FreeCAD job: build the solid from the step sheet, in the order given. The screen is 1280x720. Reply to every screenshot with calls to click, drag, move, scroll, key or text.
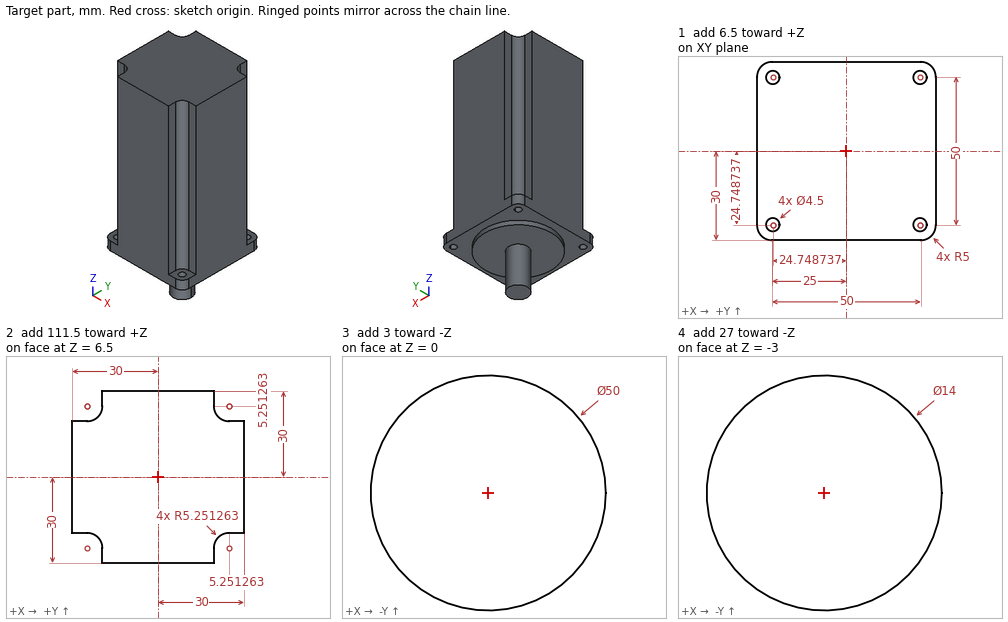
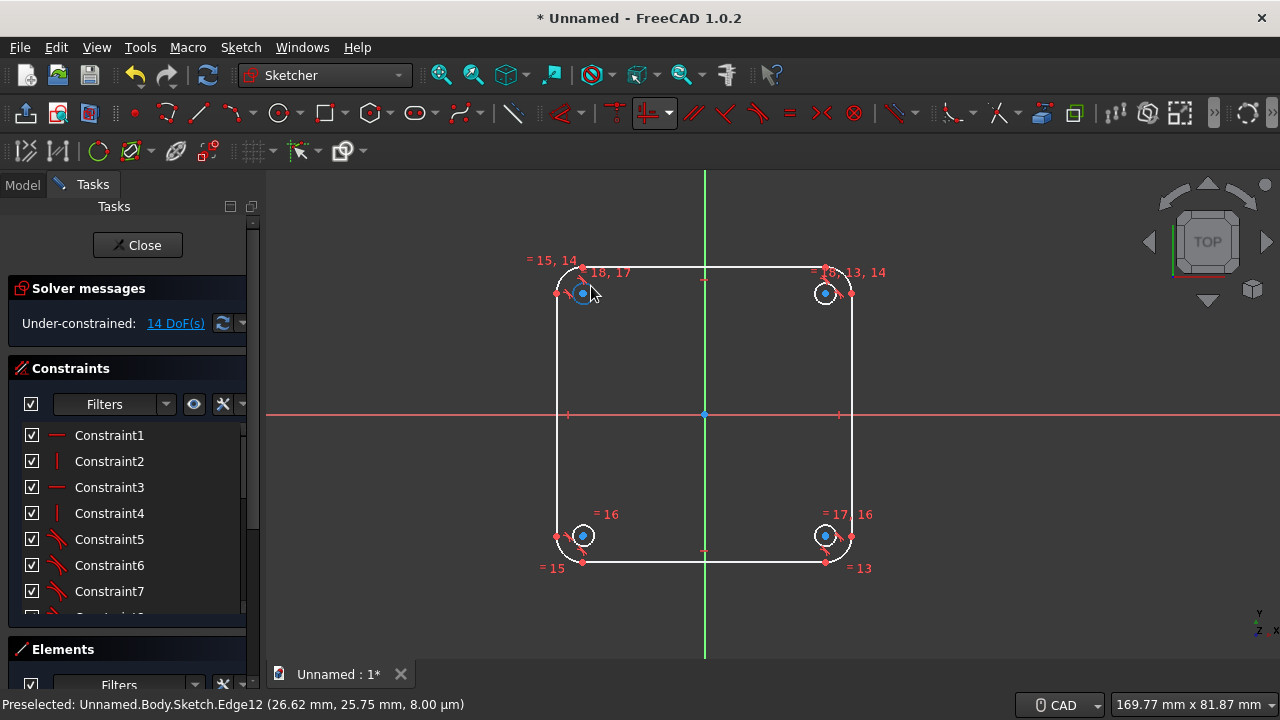
scroll(584, 536, up, 13)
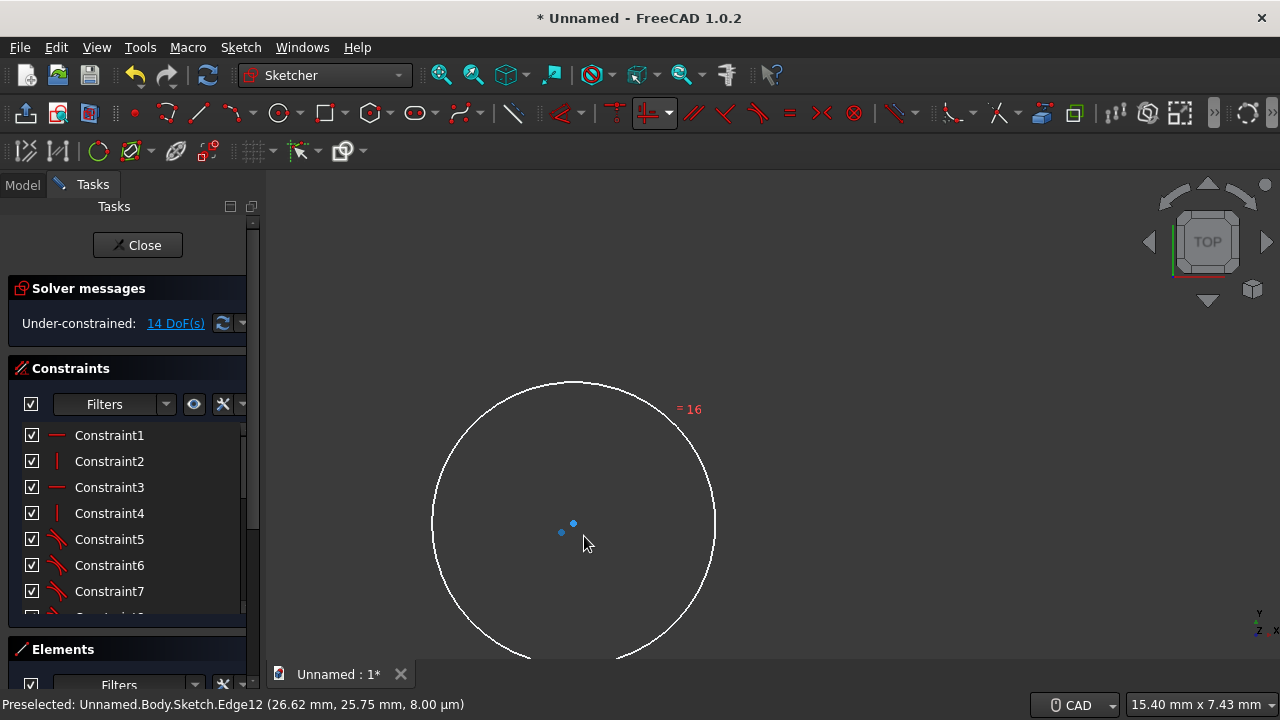
click(574, 524)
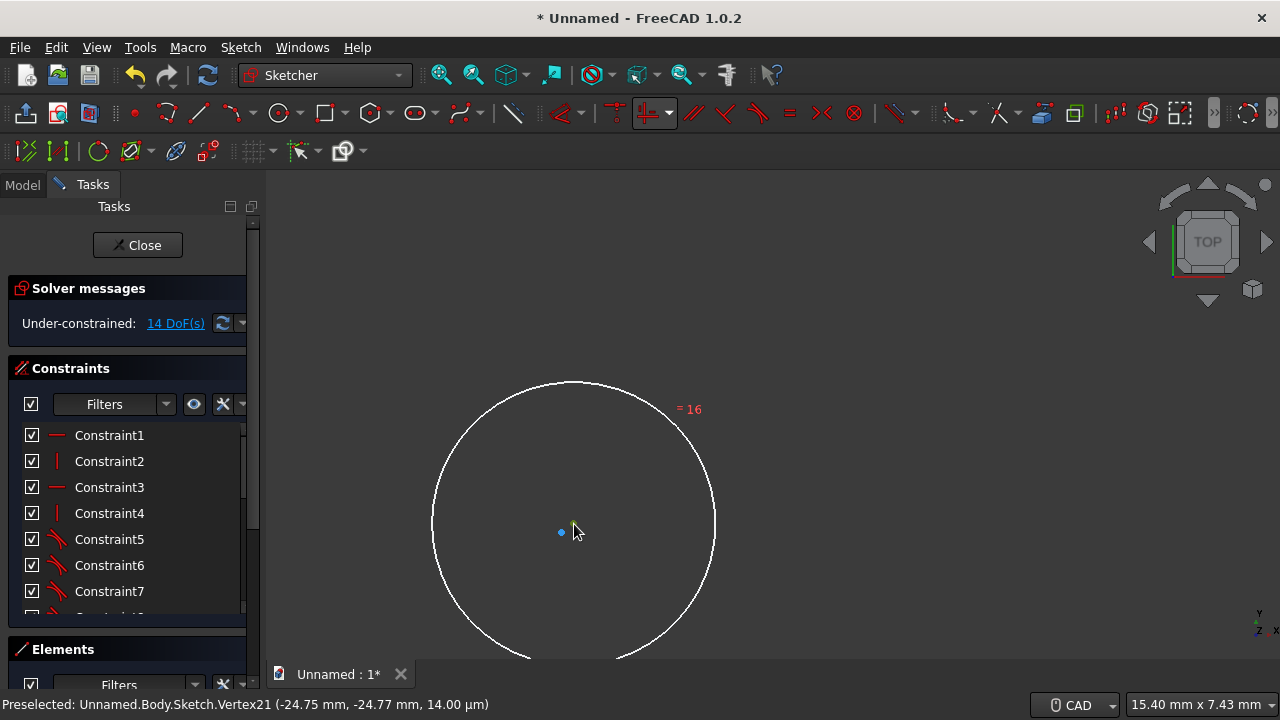
scroll(584, 537, down, 13)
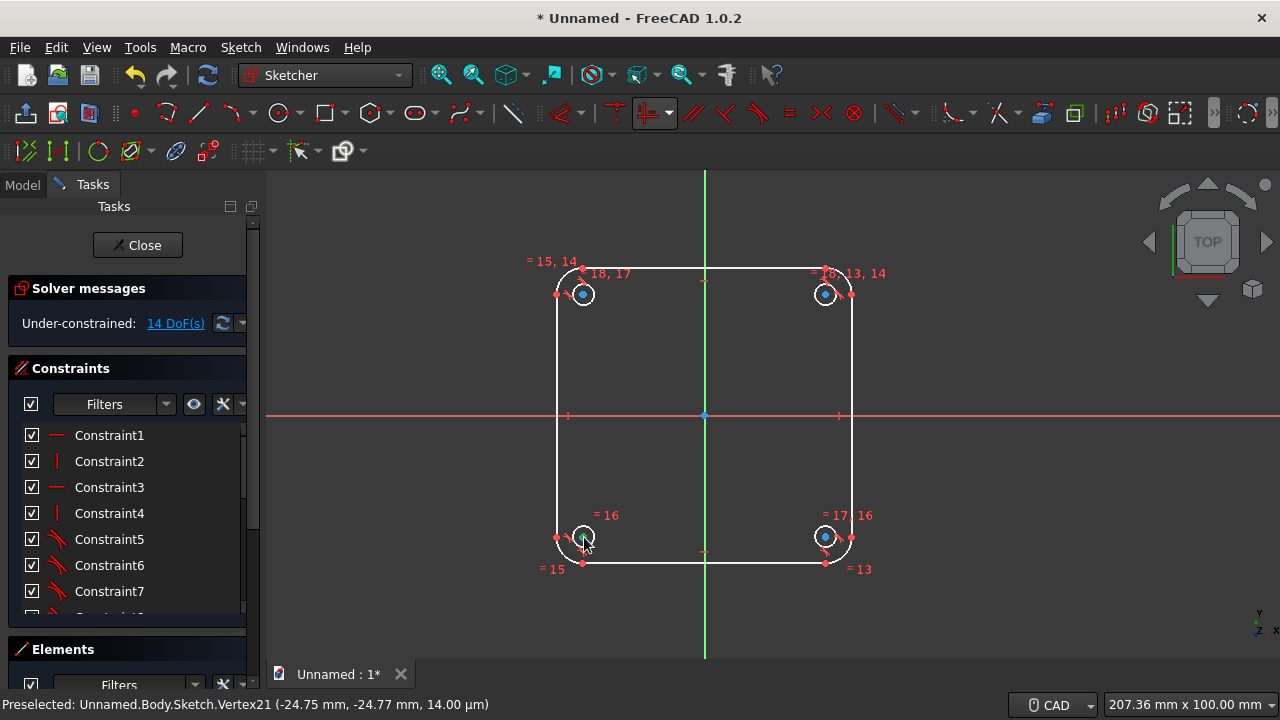
scroll(826, 537, up, 14)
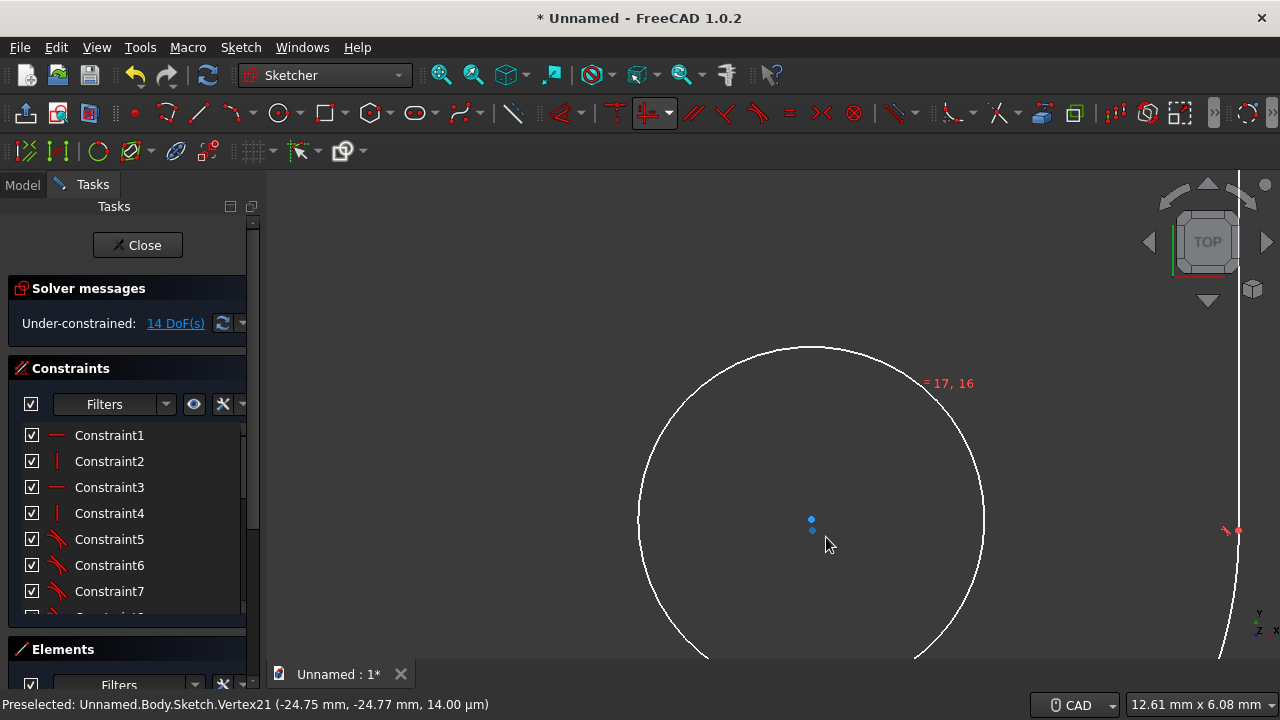
click(811, 520)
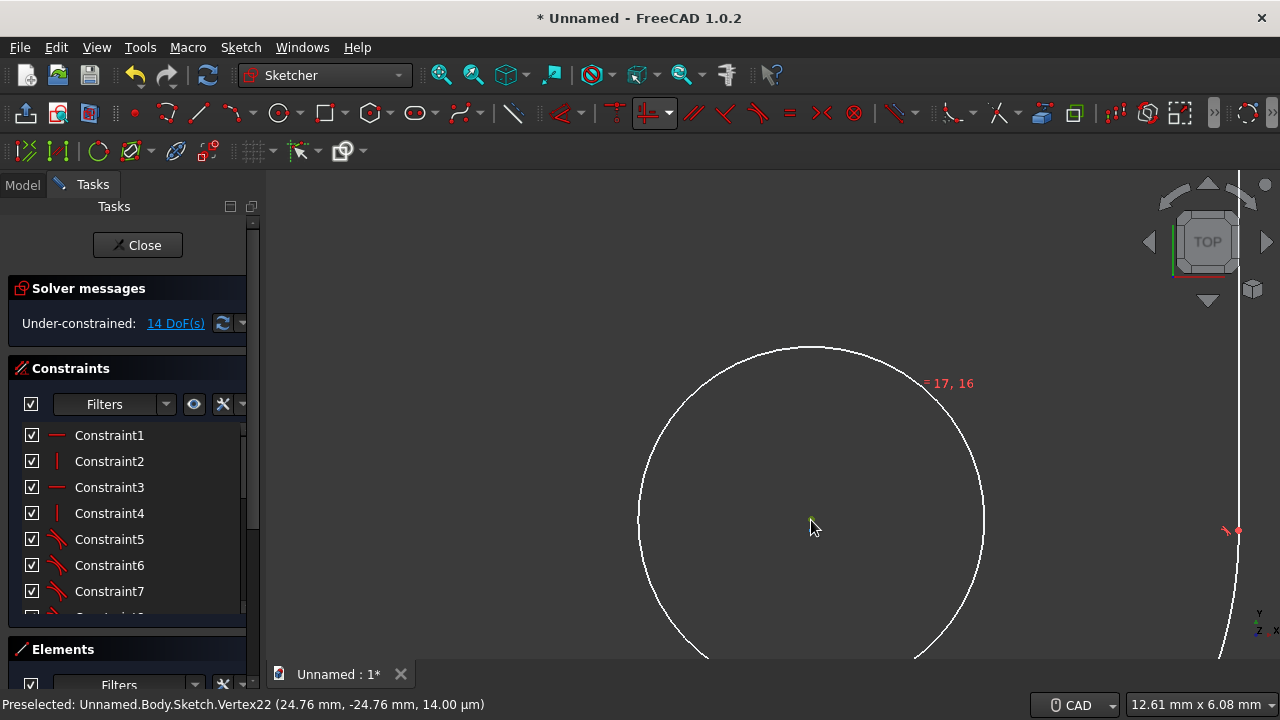
scroll(826, 537, down, 14)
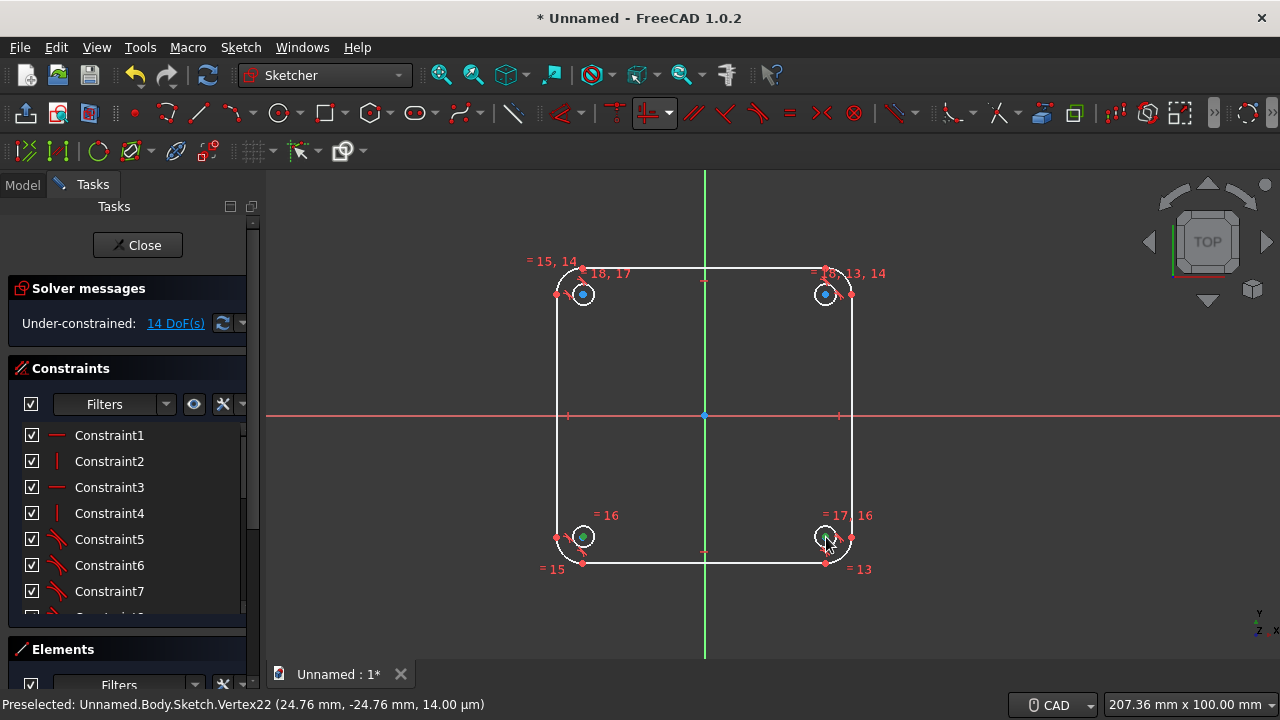
click(705, 600)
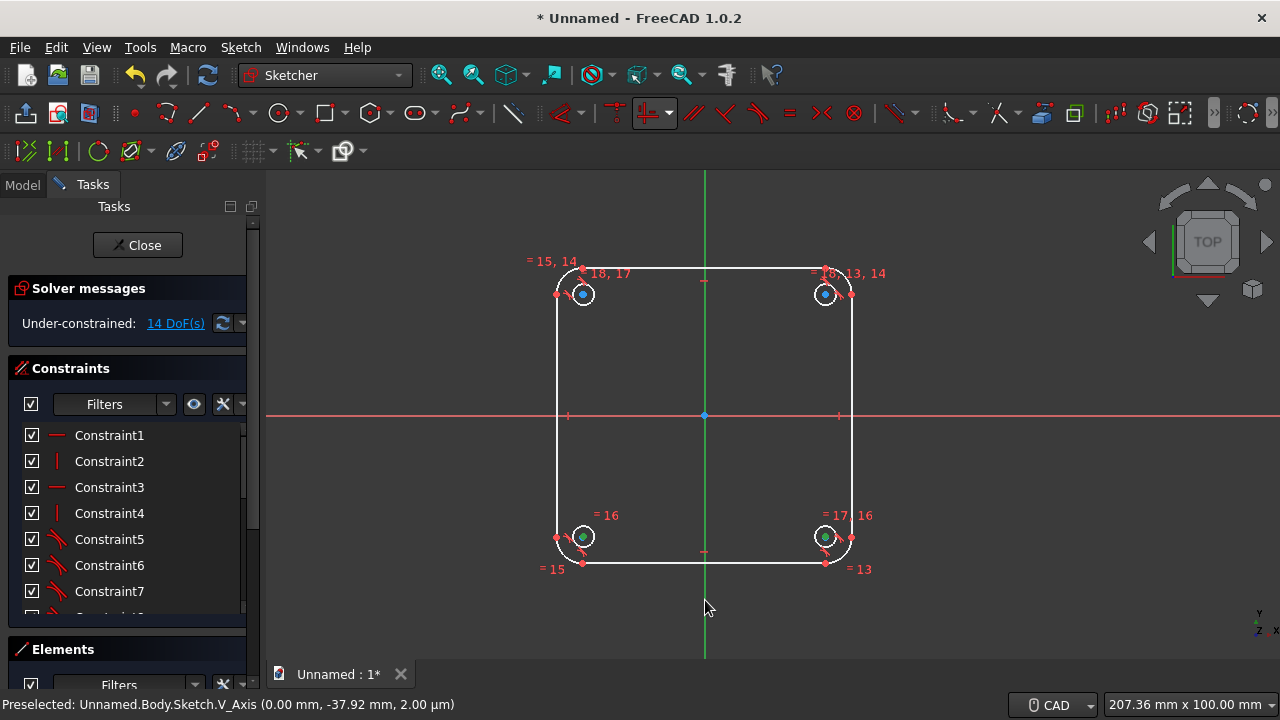
key(s)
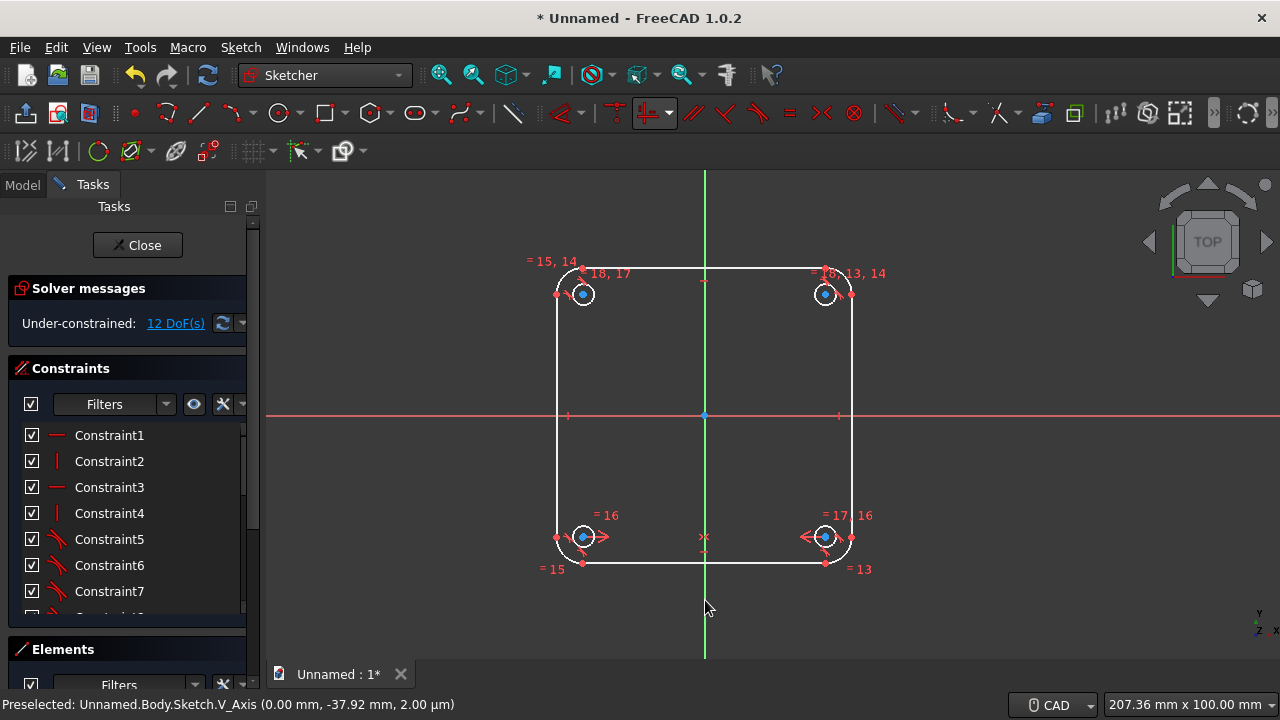
scroll(584, 537, up, 12)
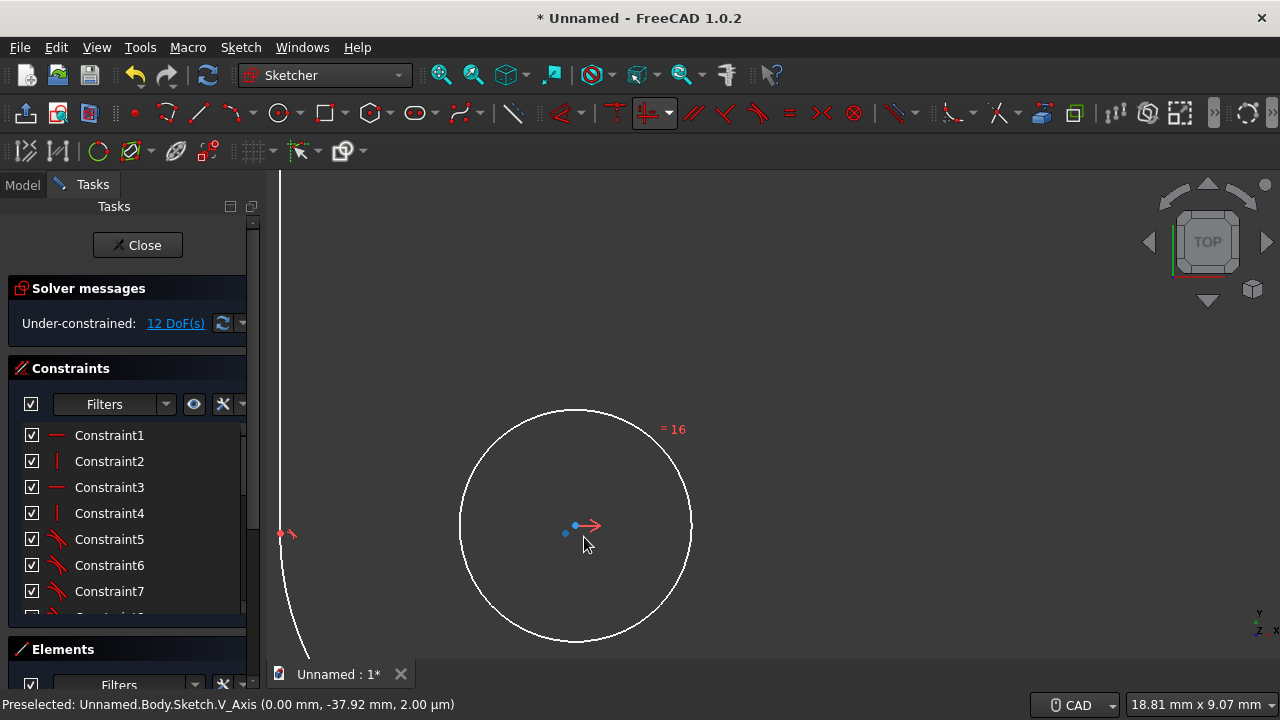
click(576, 526)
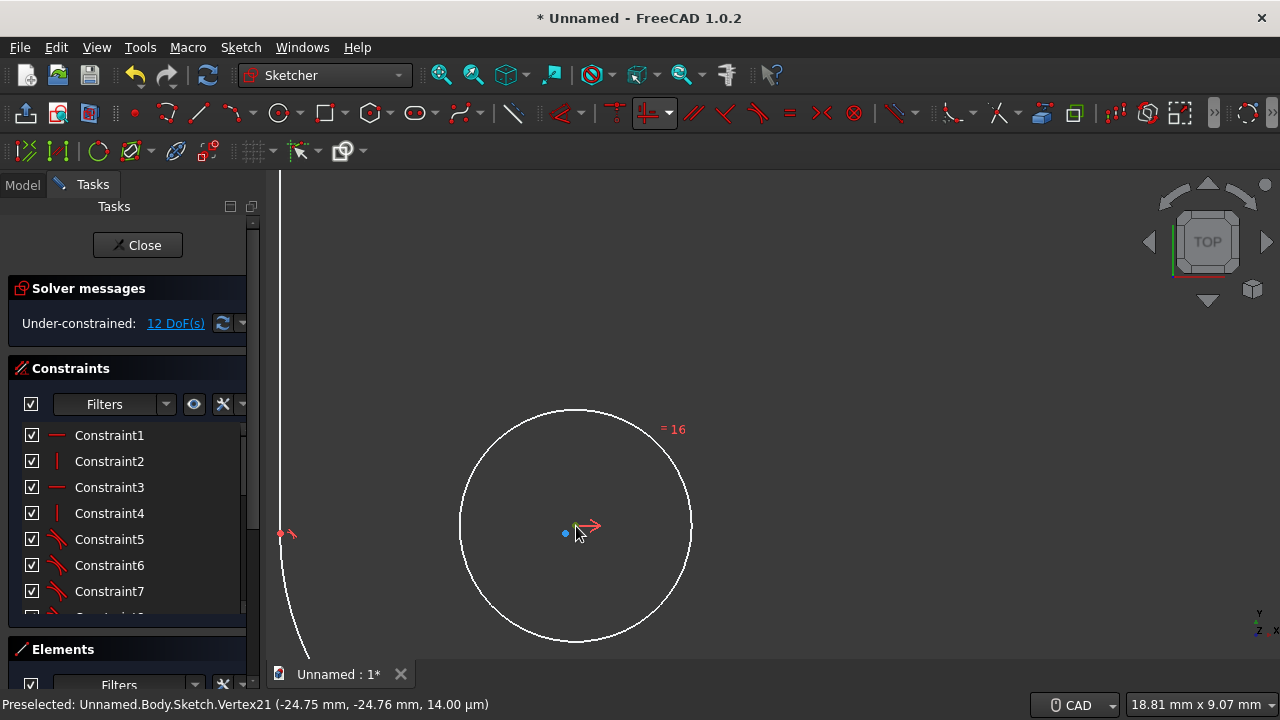
scroll(584, 537, down, 12)